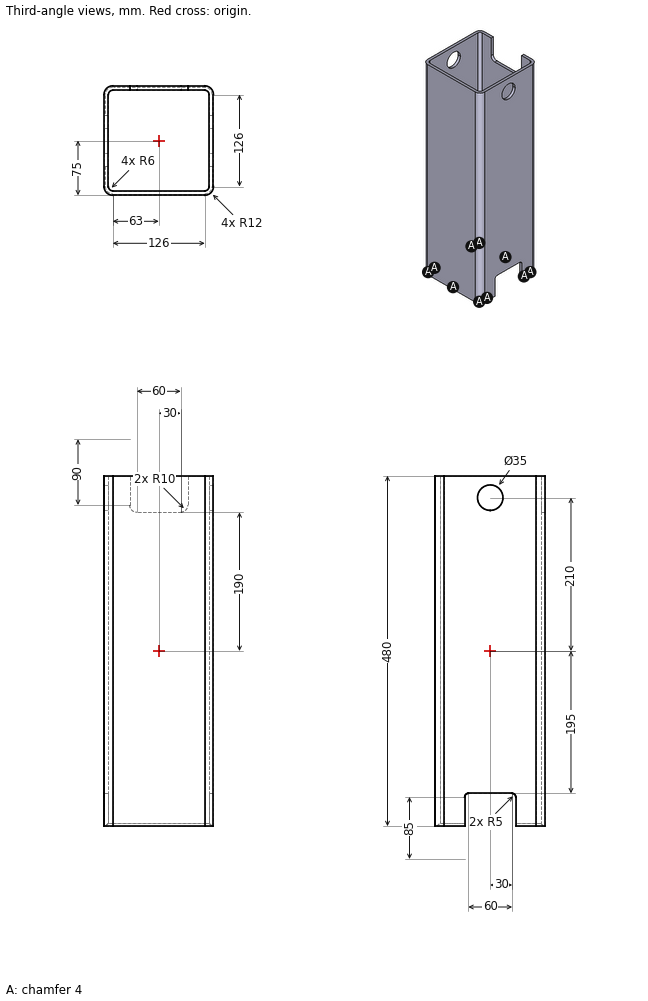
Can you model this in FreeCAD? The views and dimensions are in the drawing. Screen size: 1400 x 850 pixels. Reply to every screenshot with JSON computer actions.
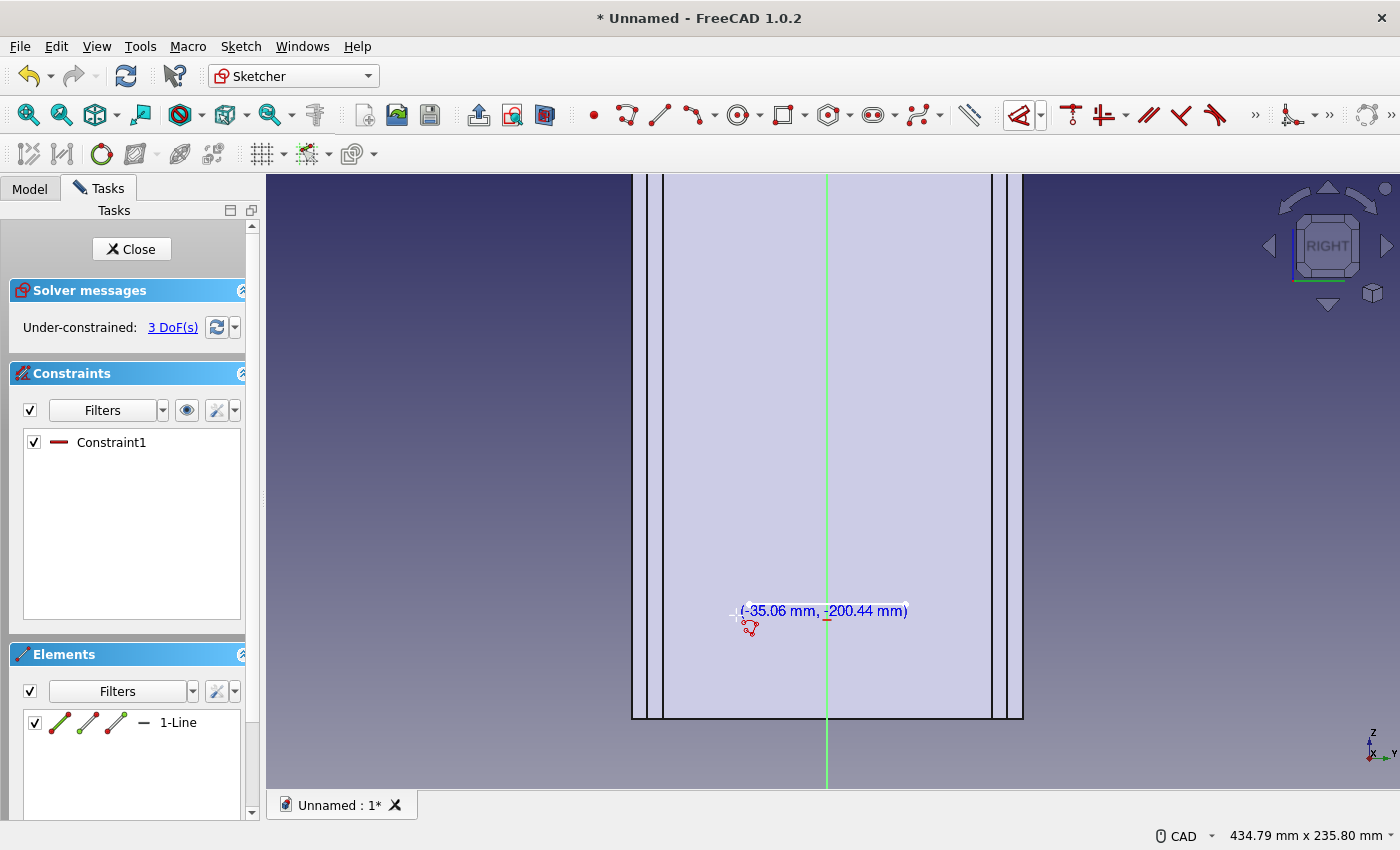
{"action": "scroll", "coordinate": [737, 617], "scroll_direction": "down", "scroll_amount": 6}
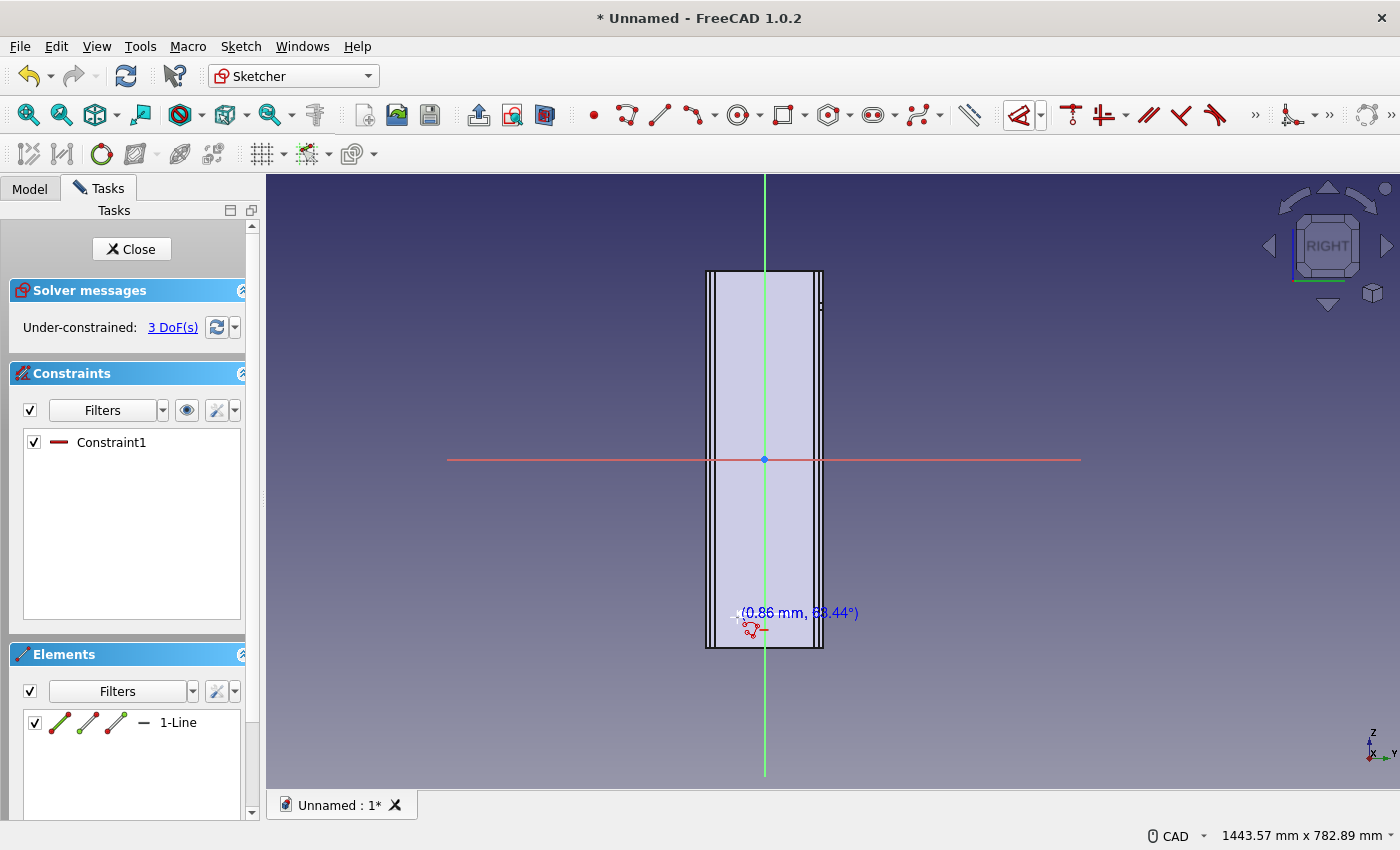
{"action": "left_click", "coordinate": [737, 684]}
{"action": "left_click", "coordinate": [792, 684]}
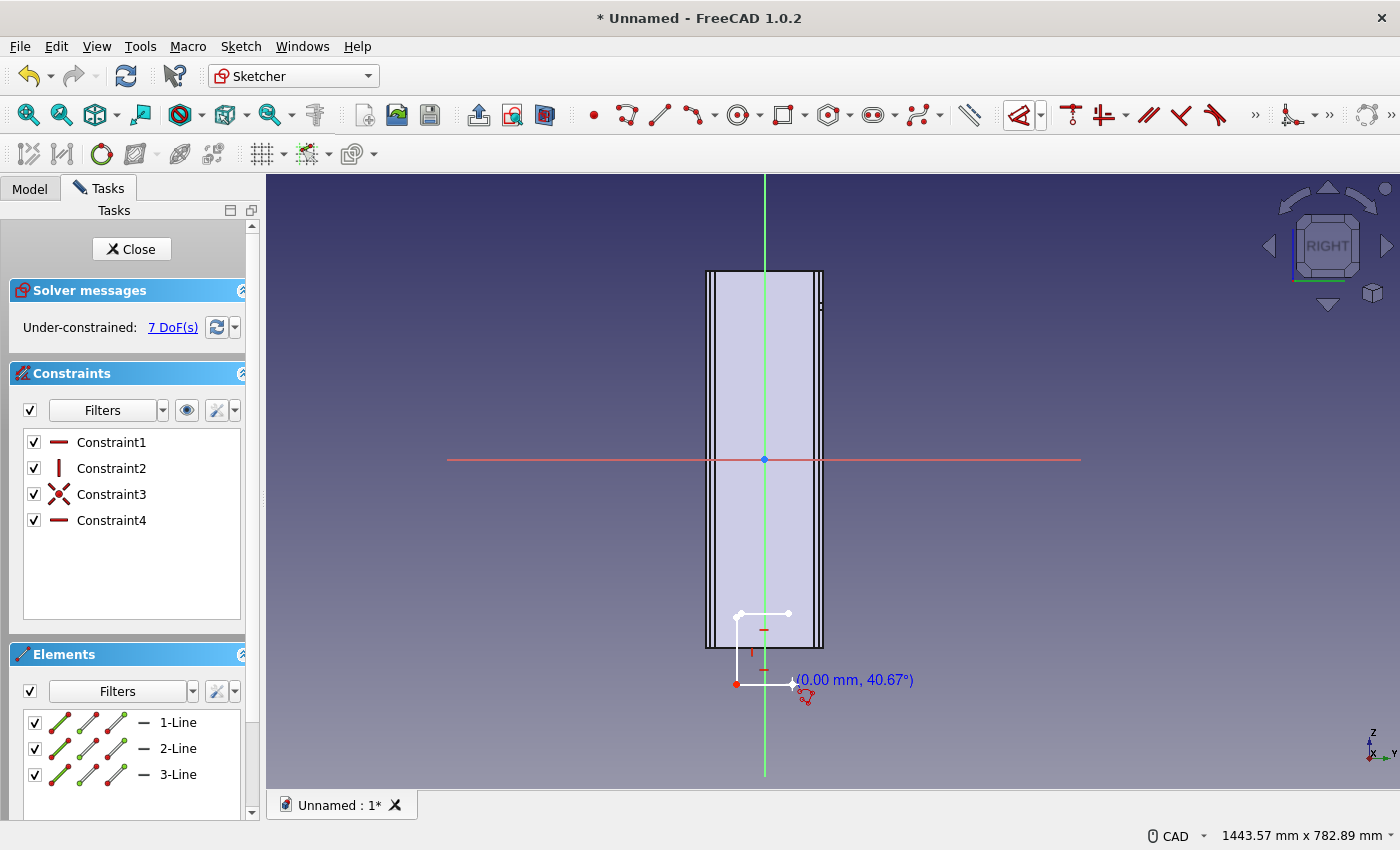
{"action": "scroll", "coordinate": [792, 617], "scroll_direction": "up", "scroll_amount": 6}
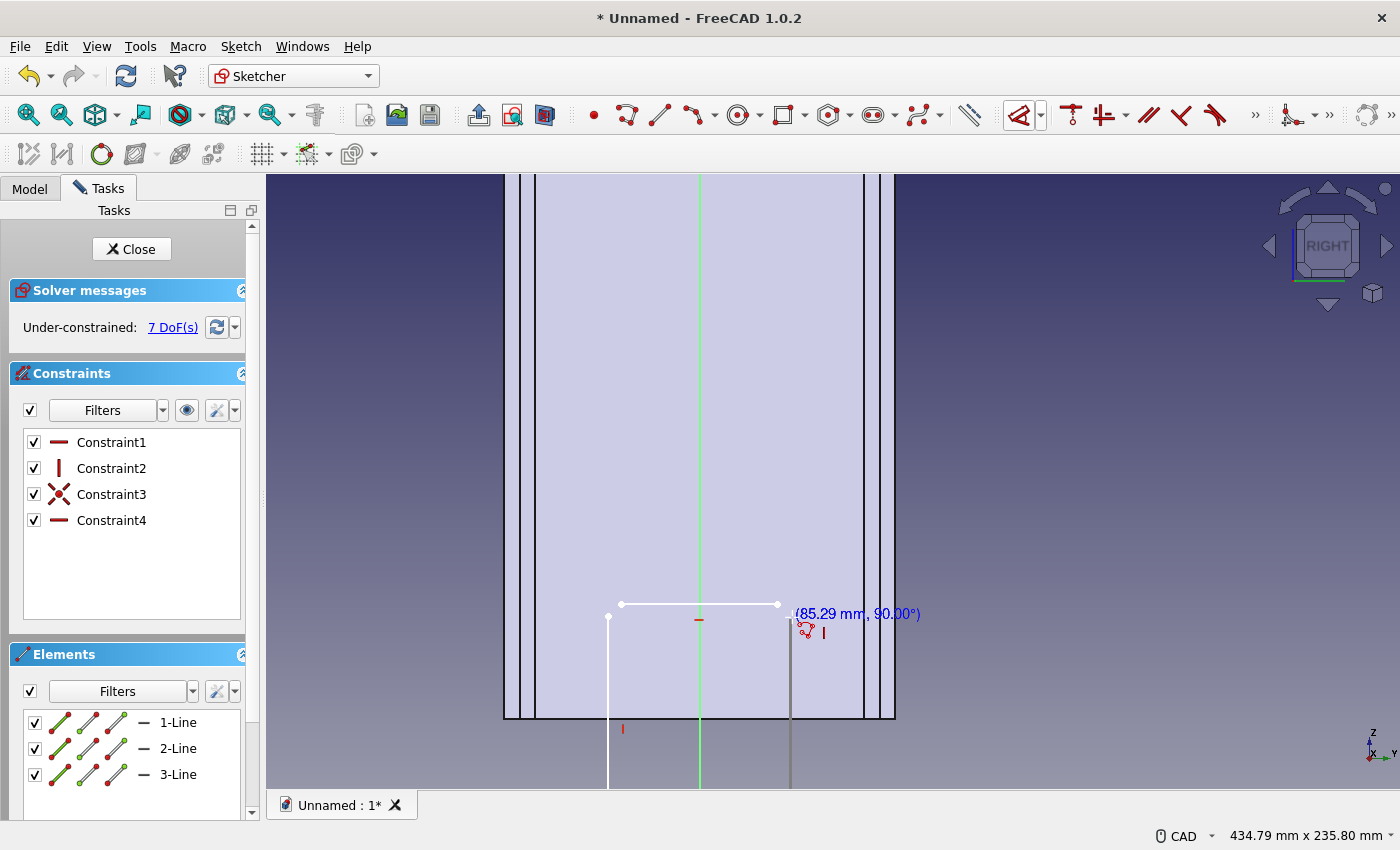
{"action": "left_click", "coordinate": [791, 615]}
{"action": "right_click", "coordinate": [791, 615]}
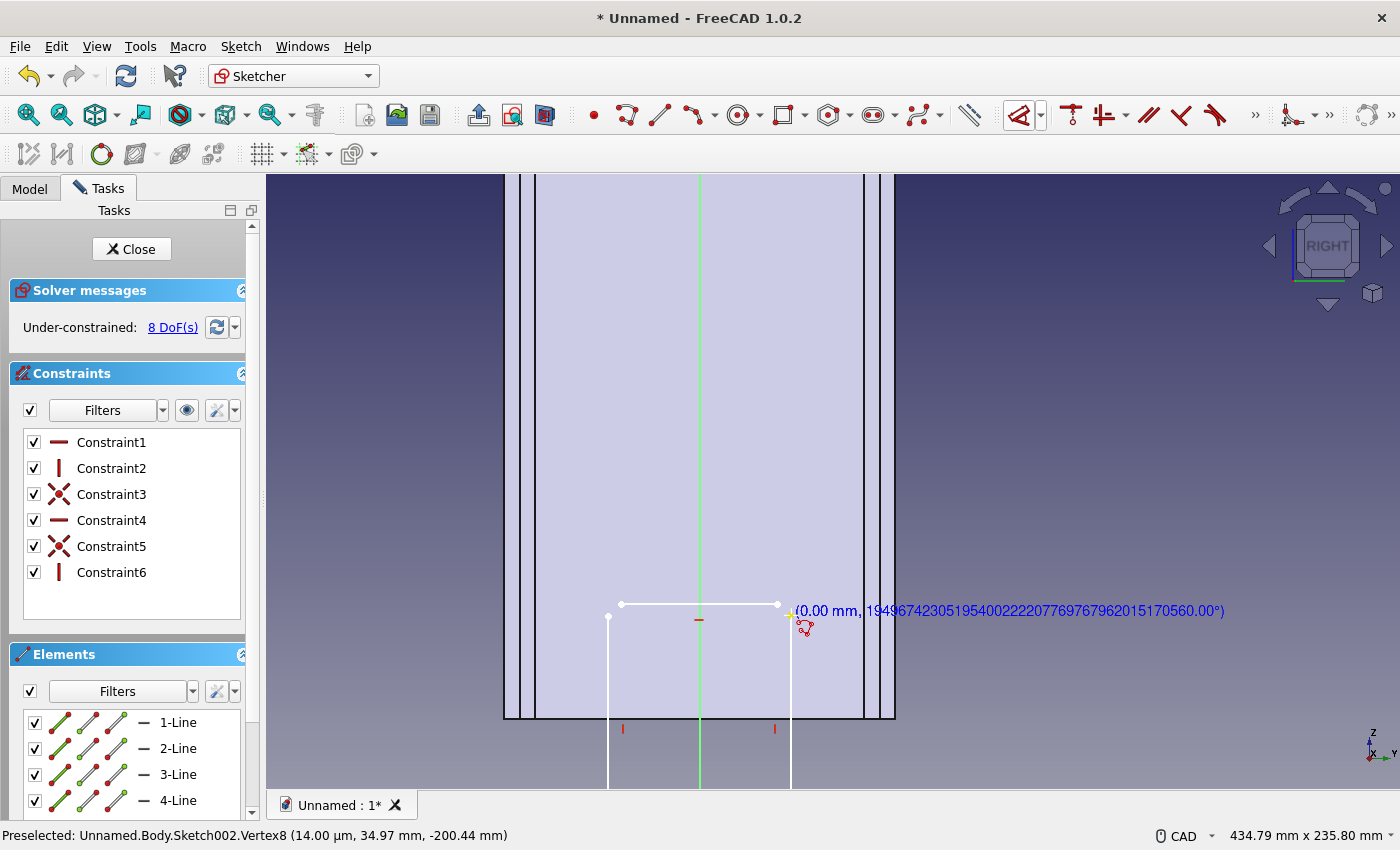
{"action": "left_click", "coordinate": [692, 116]}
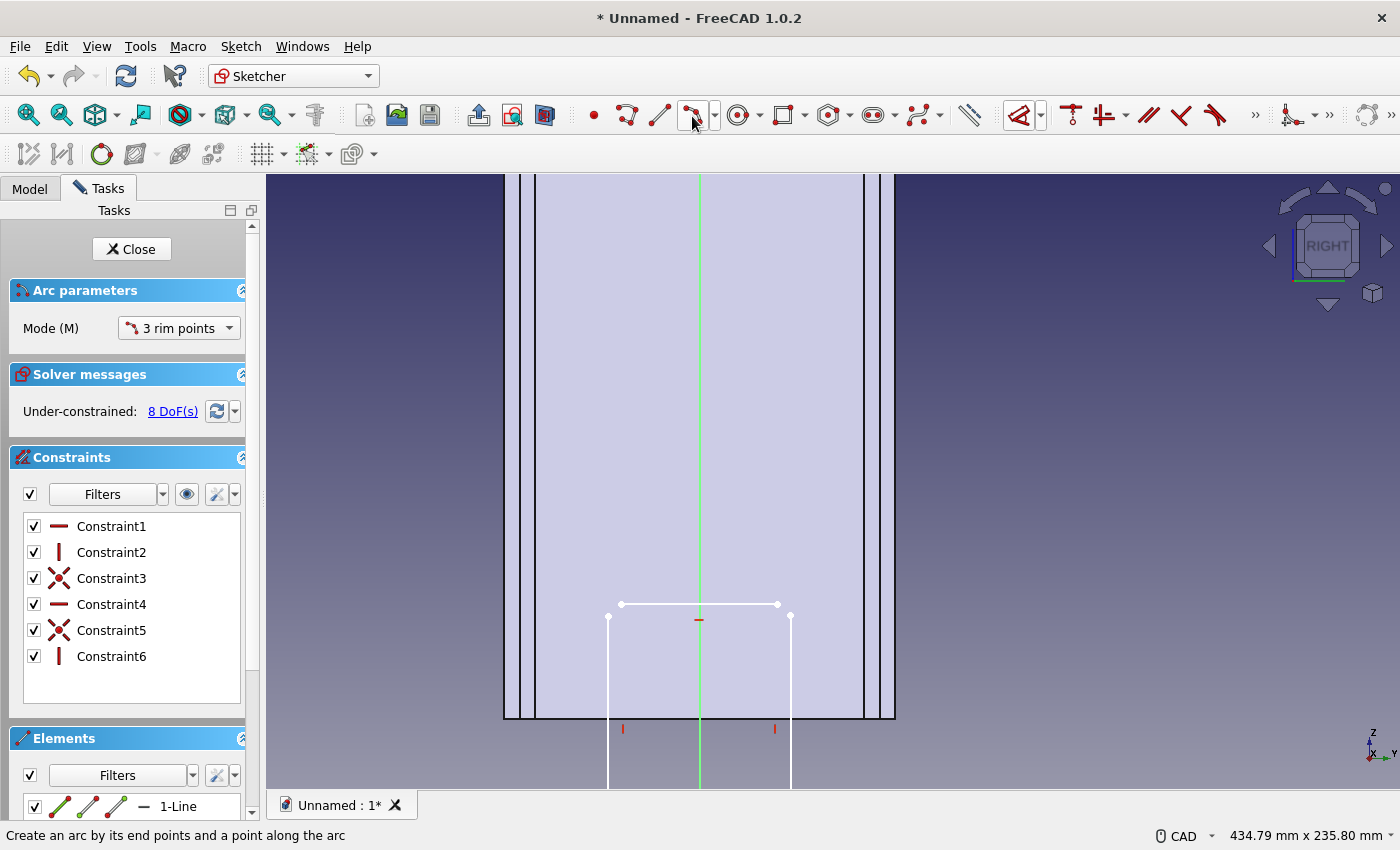
{"action": "left_click", "coordinate": [622, 604]}
{"action": "left_click", "coordinate": [608, 616]}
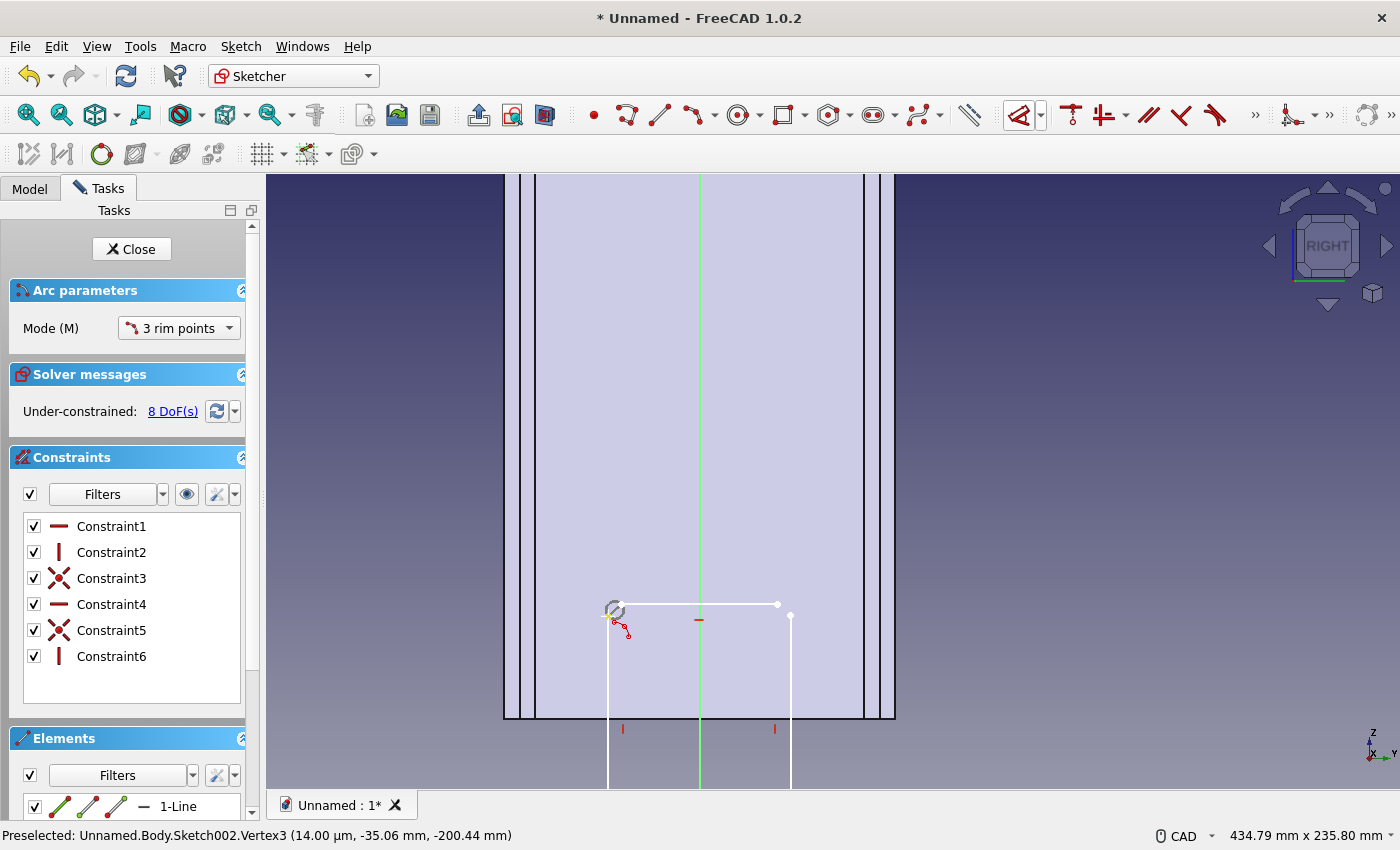
{"action": "scroll", "coordinate": [612, 606], "scroll_direction": "up", "scroll_amount": 8}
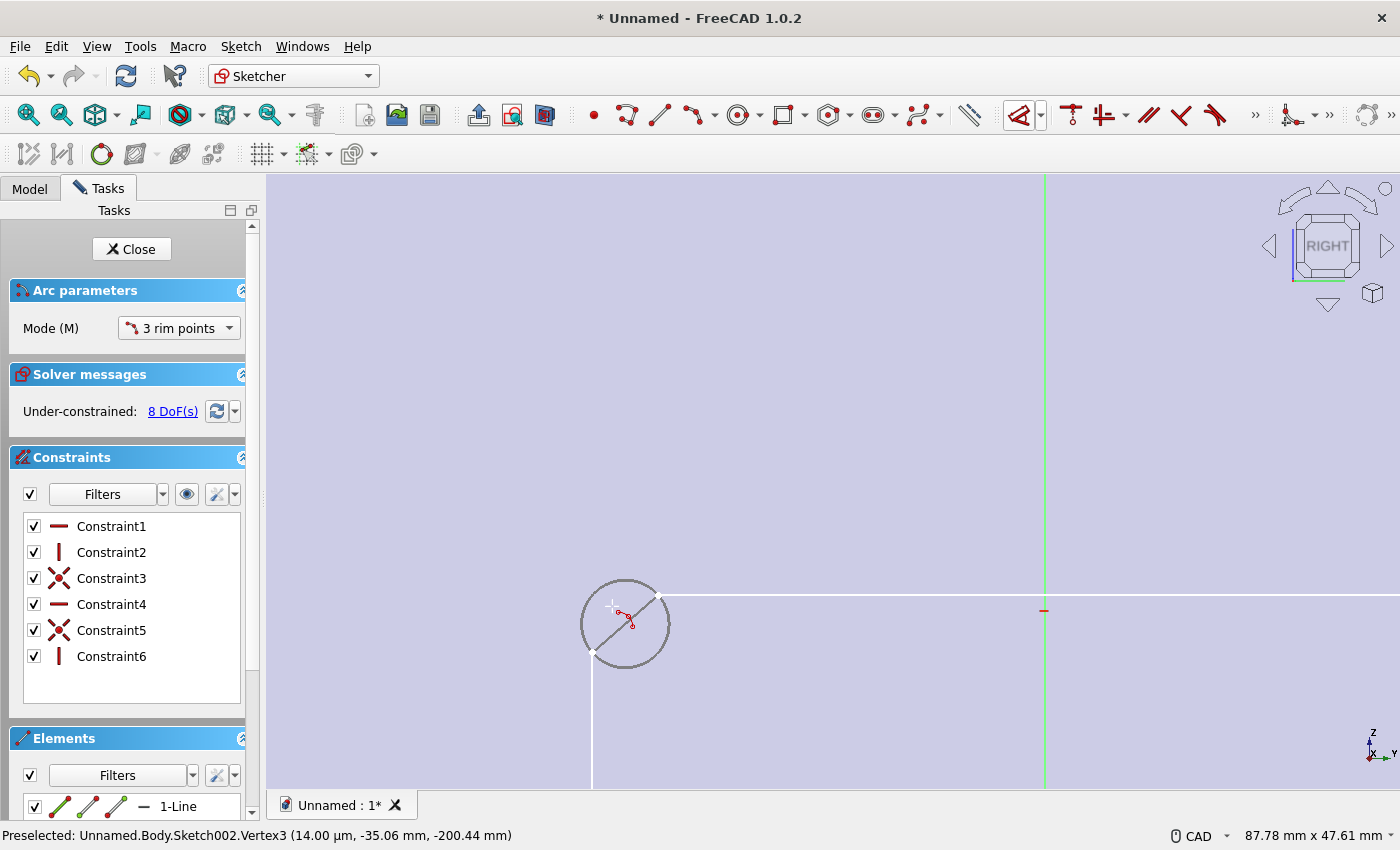
{"action": "left_click", "coordinate": [612, 601]}